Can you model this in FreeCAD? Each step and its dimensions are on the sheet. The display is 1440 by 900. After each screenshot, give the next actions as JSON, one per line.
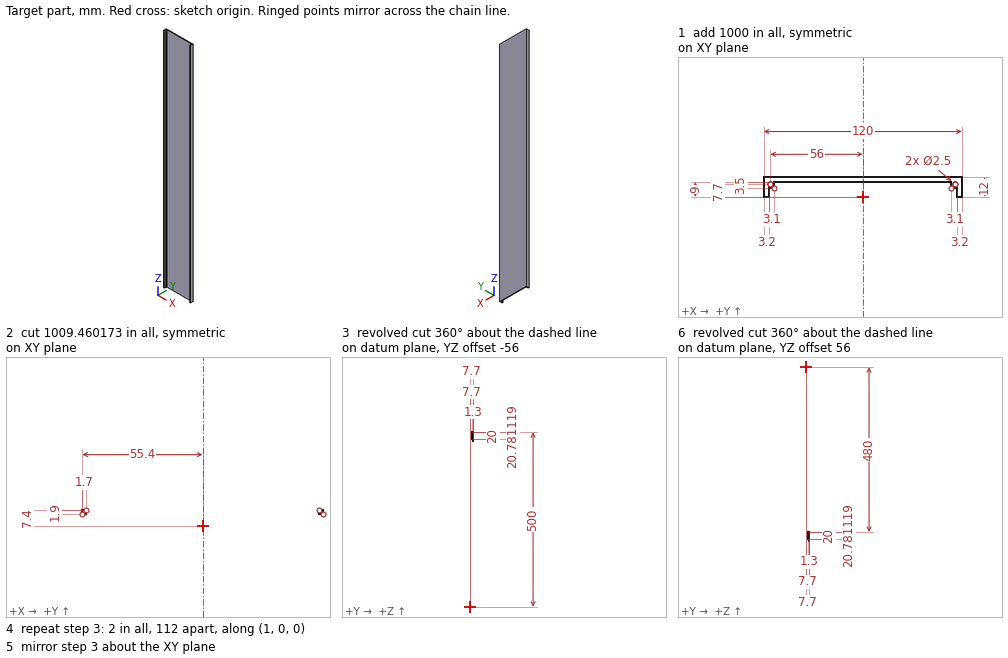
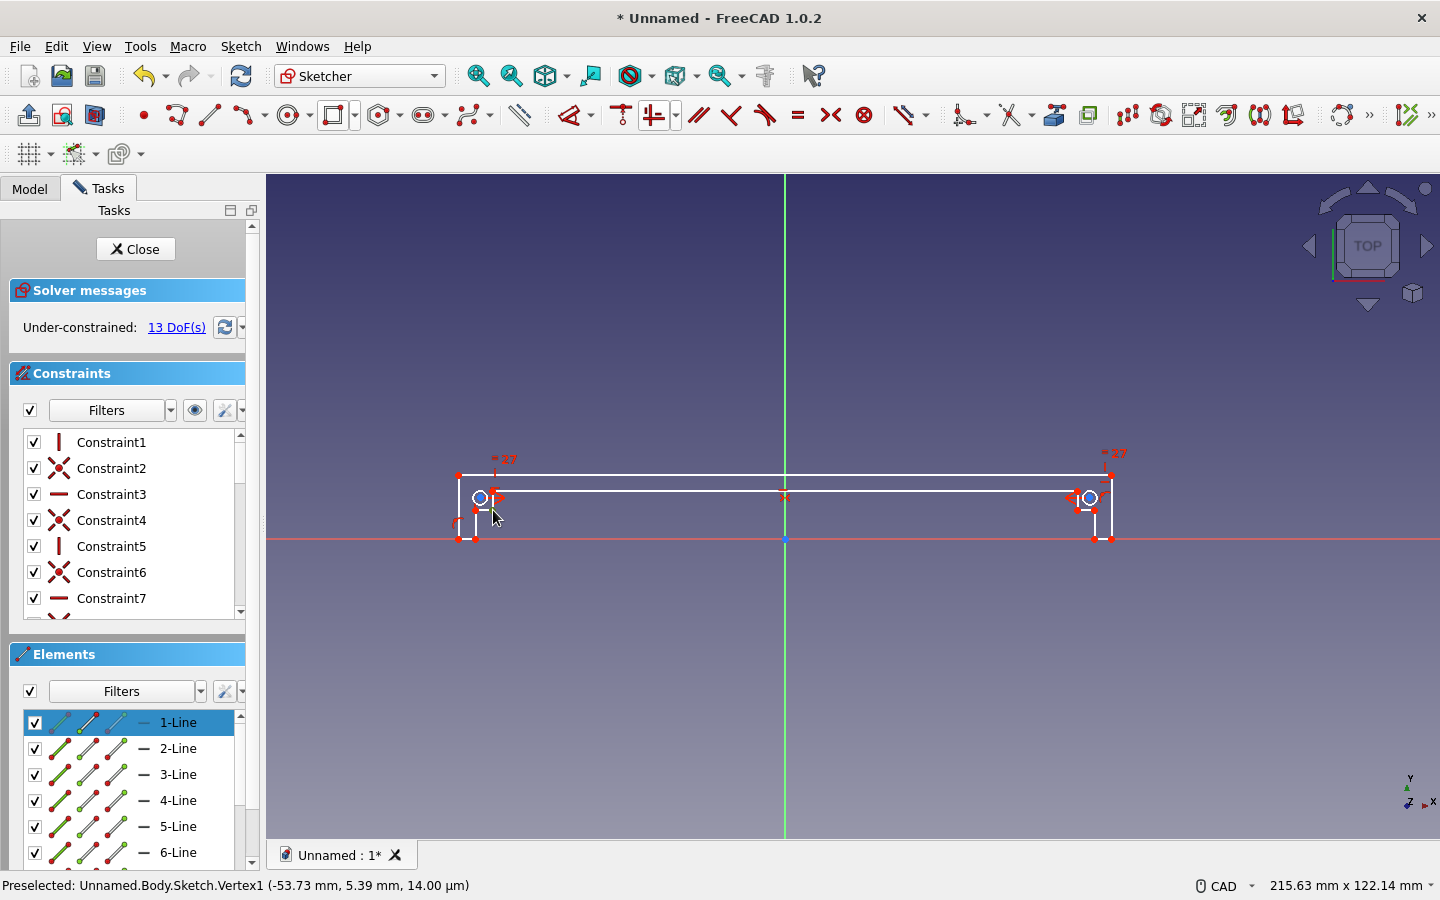
{"action": "left_click", "coordinate": [1078, 510]}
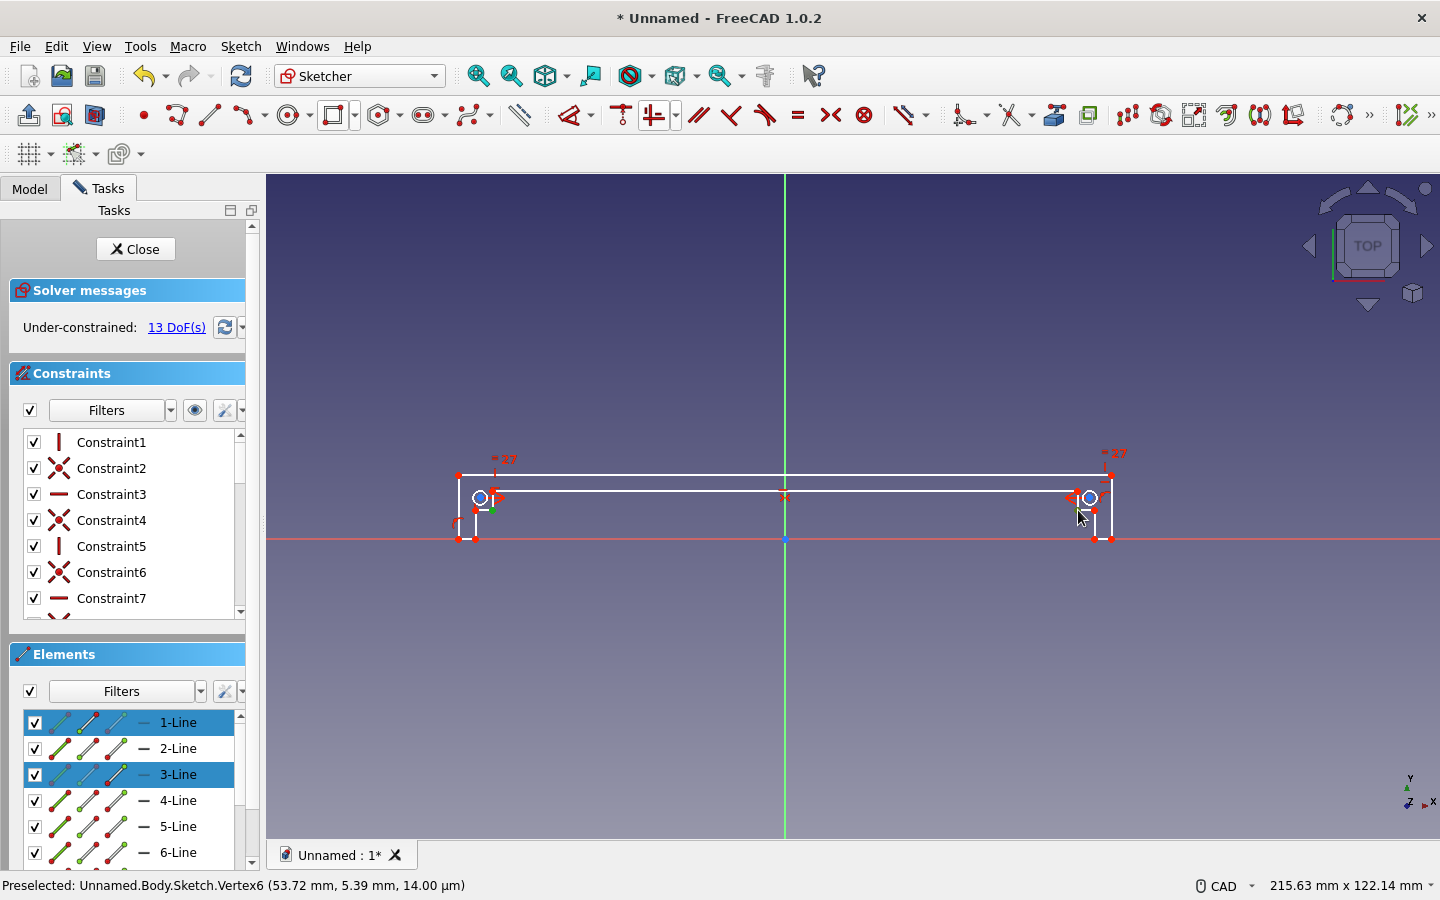
{"action": "left_click", "coordinate": [785, 768]}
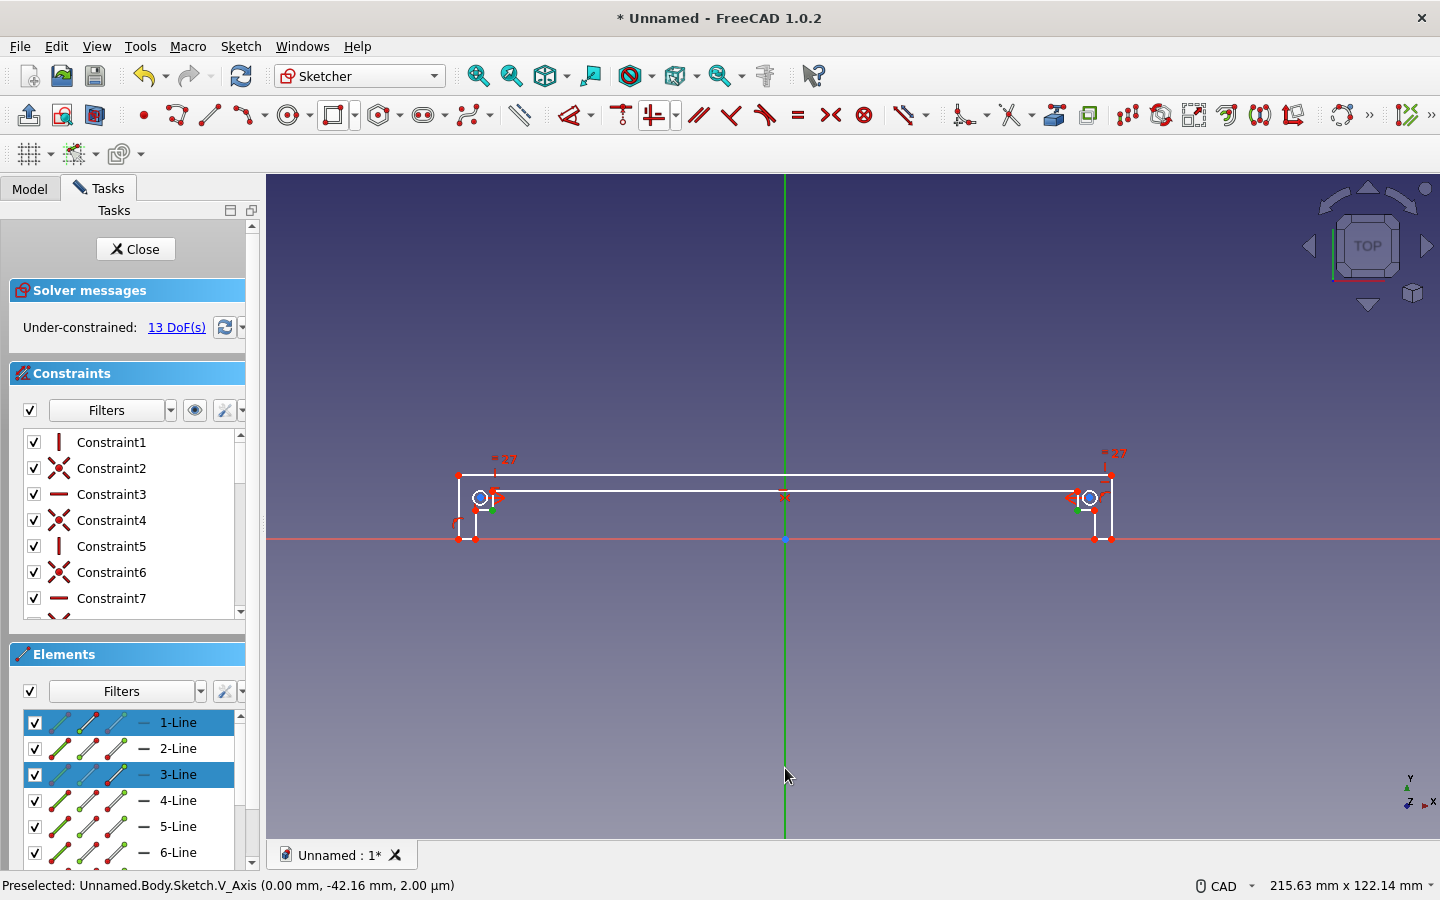
{"action": "key", "text": "s"}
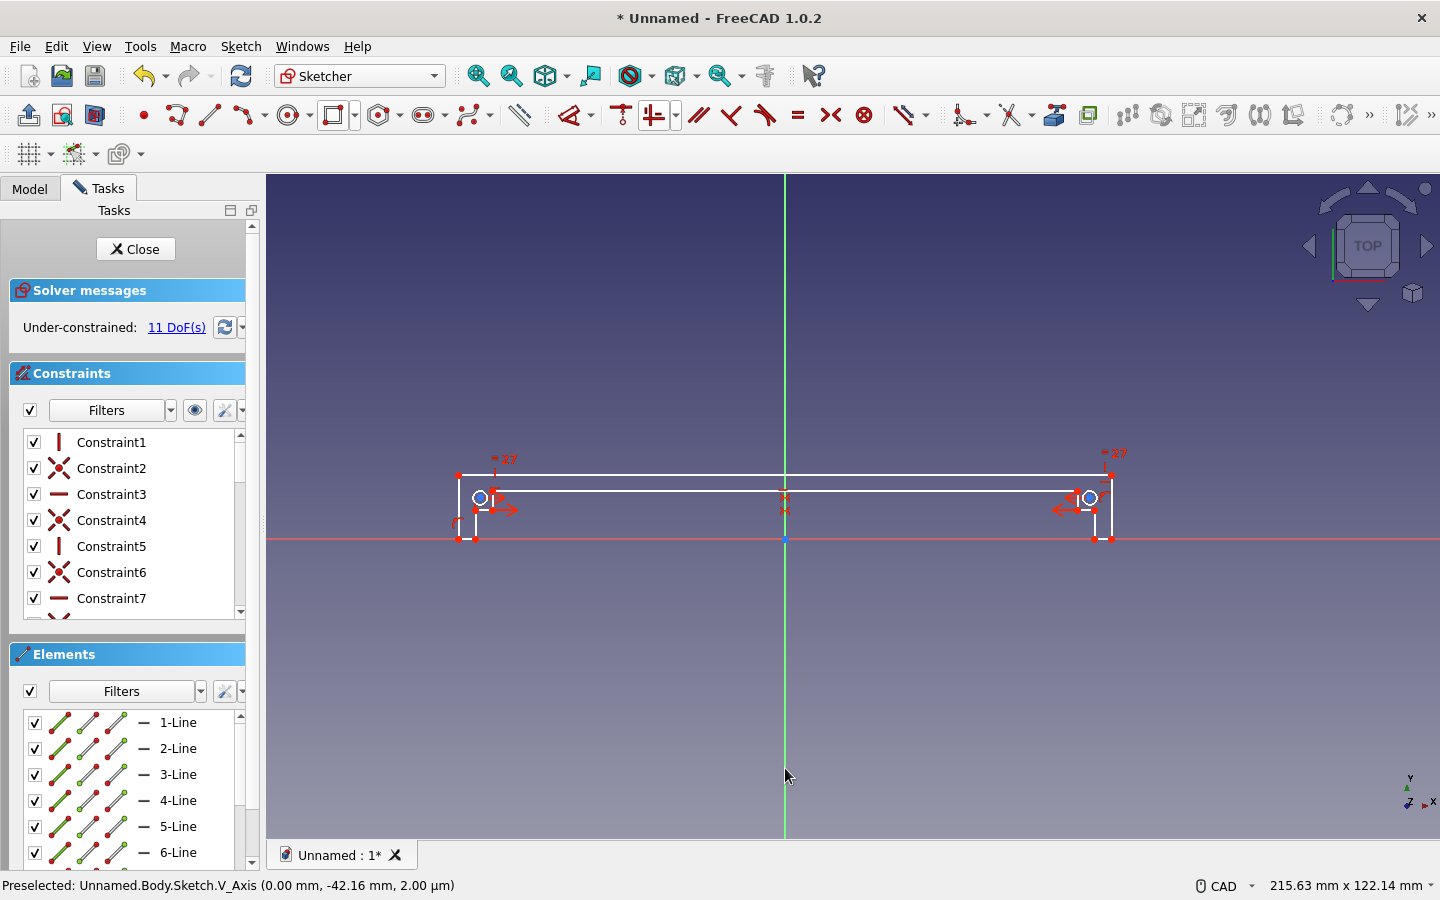
{"action": "key", "text": "d"}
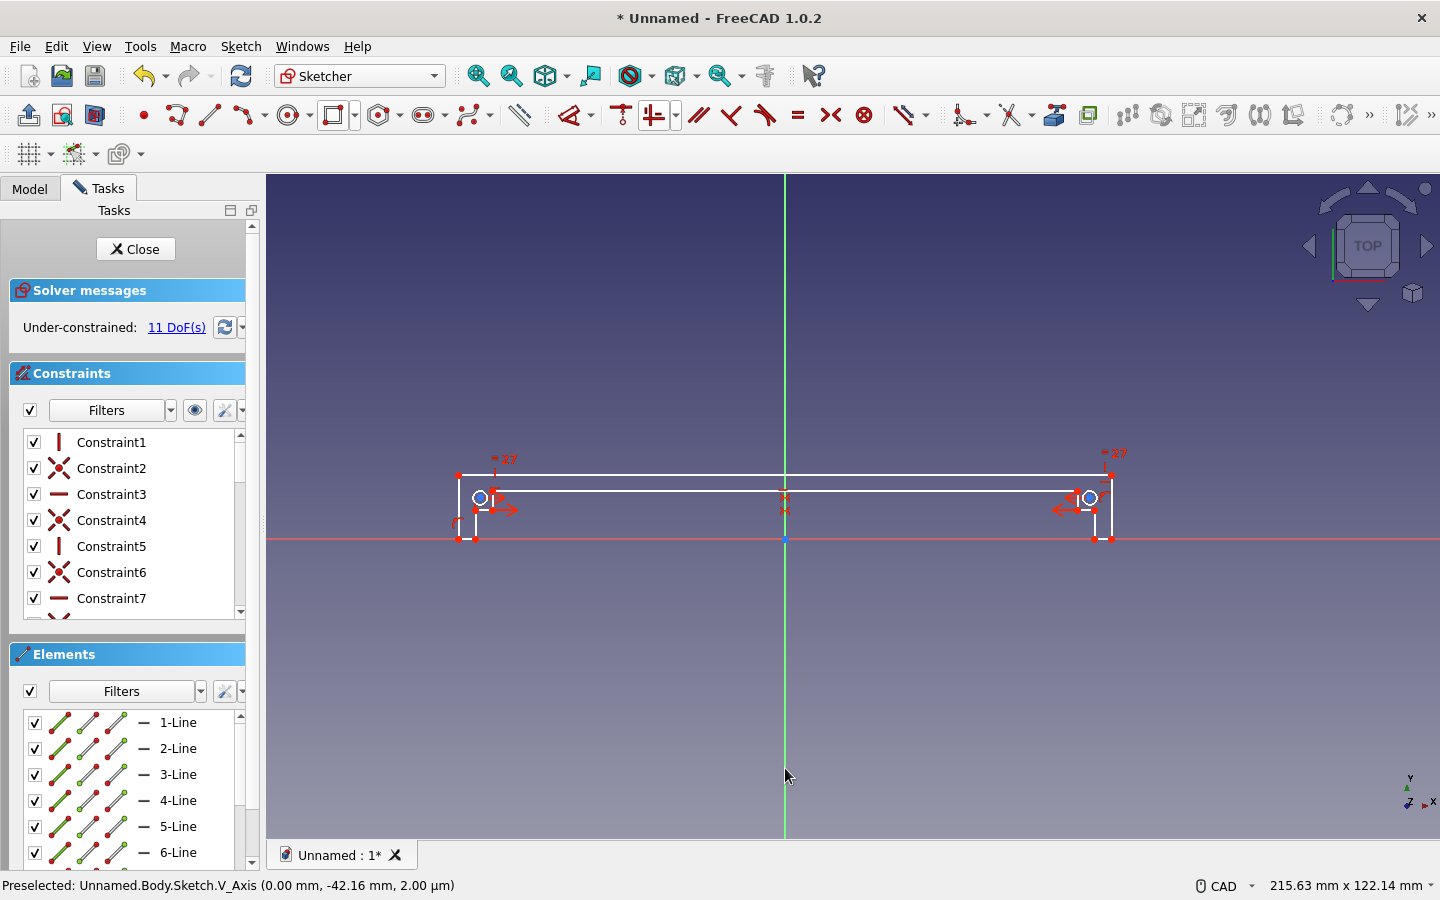
{"action": "scroll", "coordinate": [485, 503], "scroll_direction": "up", "scroll_amount": 6}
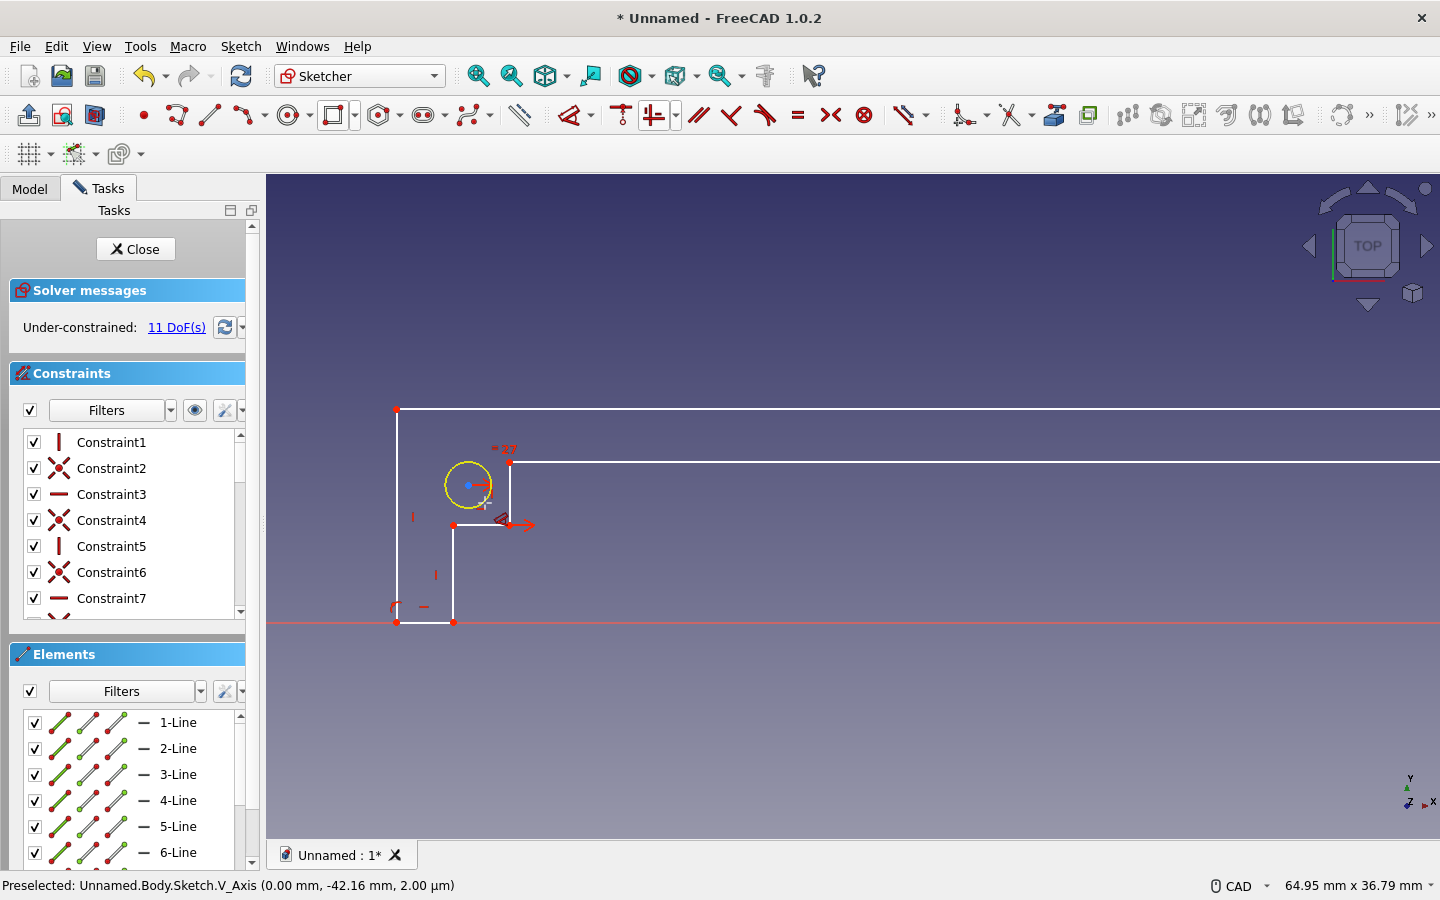
{"action": "left_click", "coordinate": [485, 501]}
{"action": "left_click", "coordinate": [430, 525]}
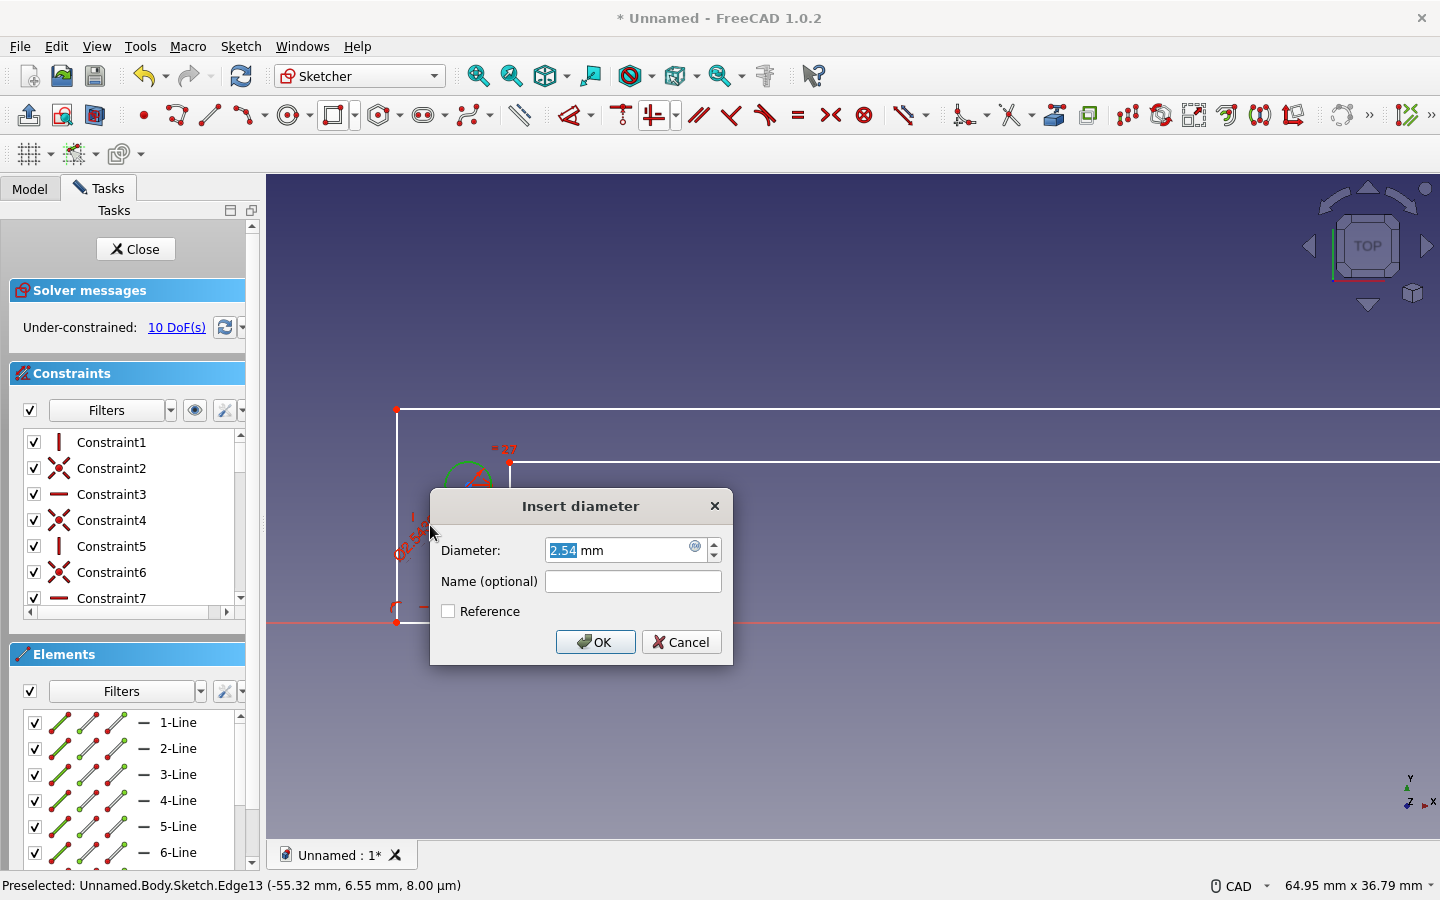
{"action": "type", "text": "2.5"}
{"action": "key", "text": "Return"}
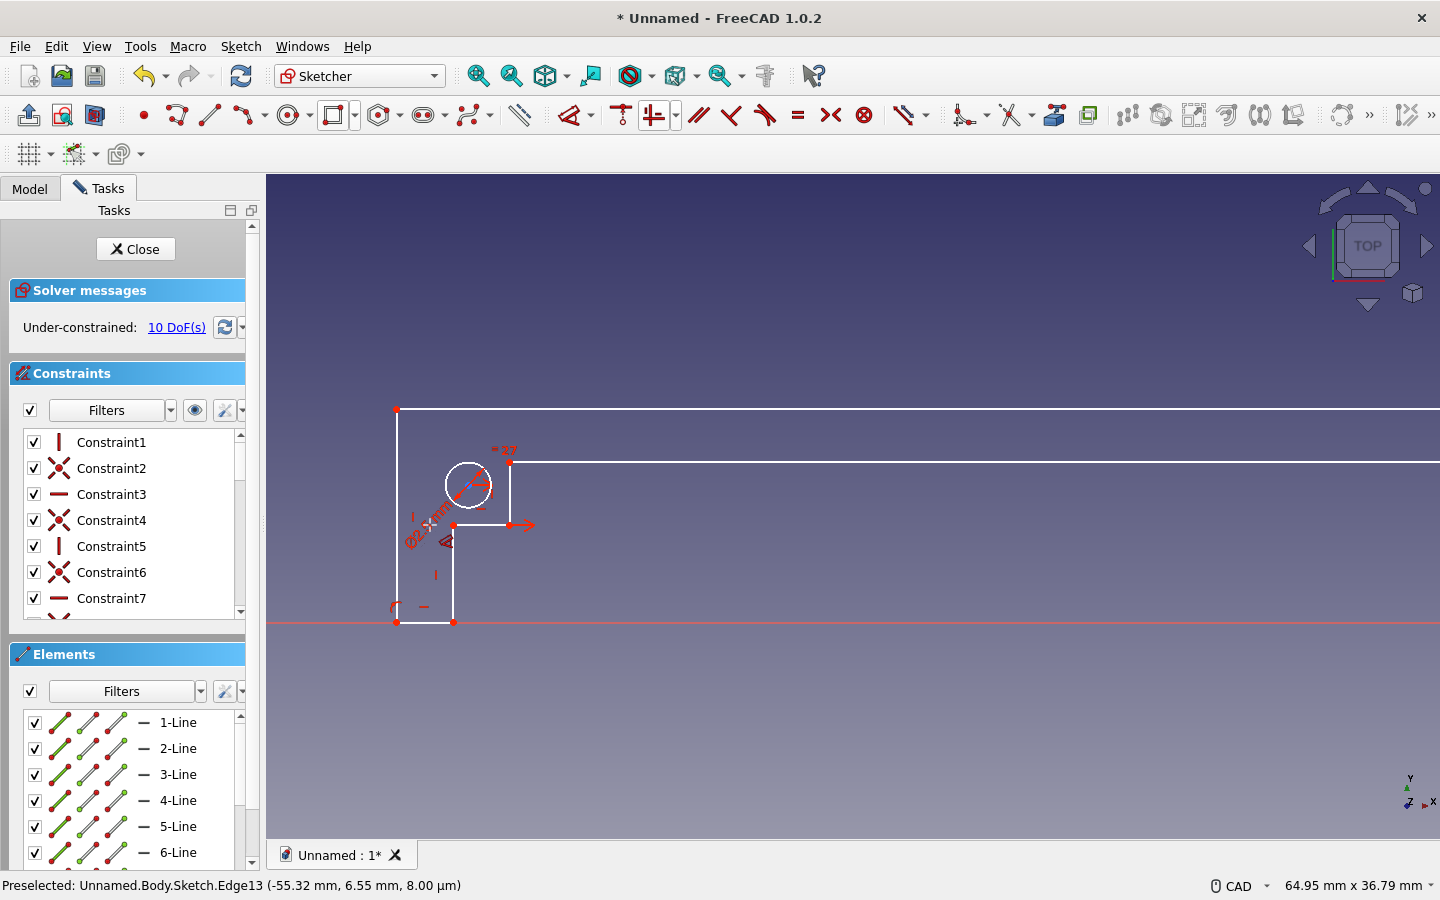
{"action": "scroll", "coordinate": [484, 503], "scroll_direction": "down", "scroll_amount": 6}